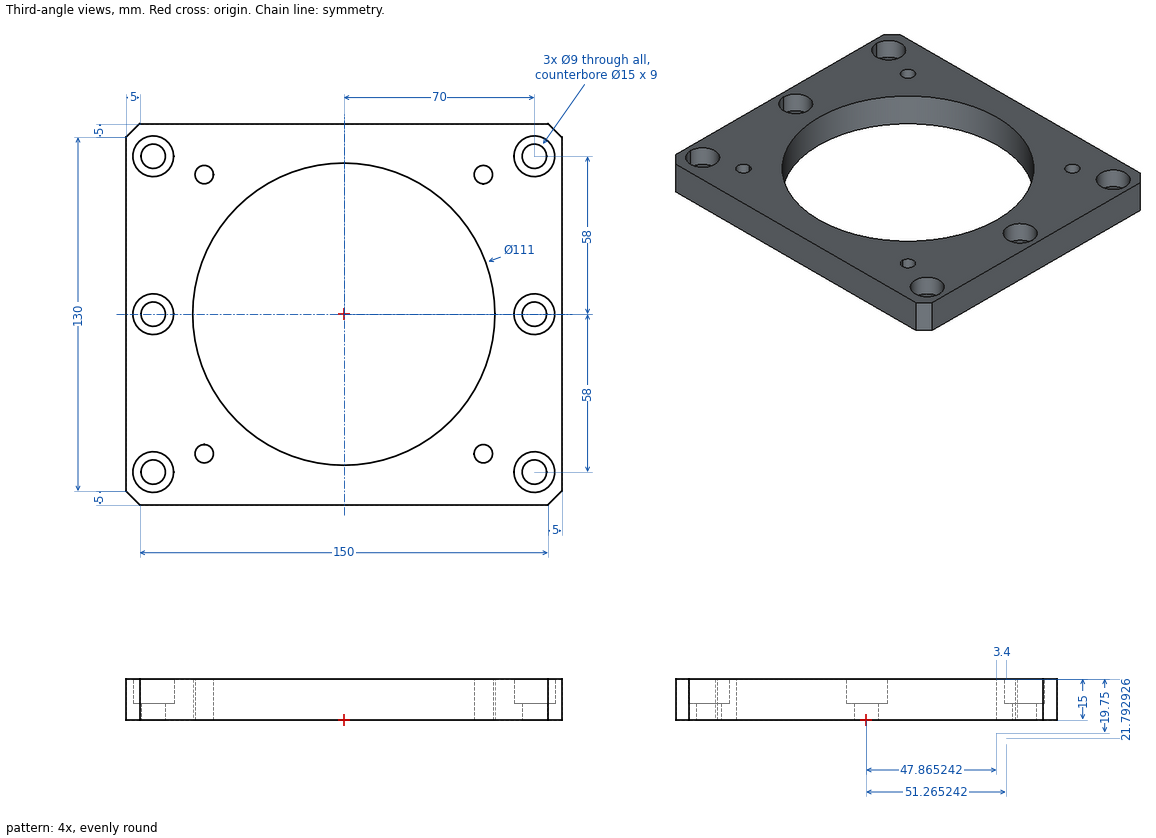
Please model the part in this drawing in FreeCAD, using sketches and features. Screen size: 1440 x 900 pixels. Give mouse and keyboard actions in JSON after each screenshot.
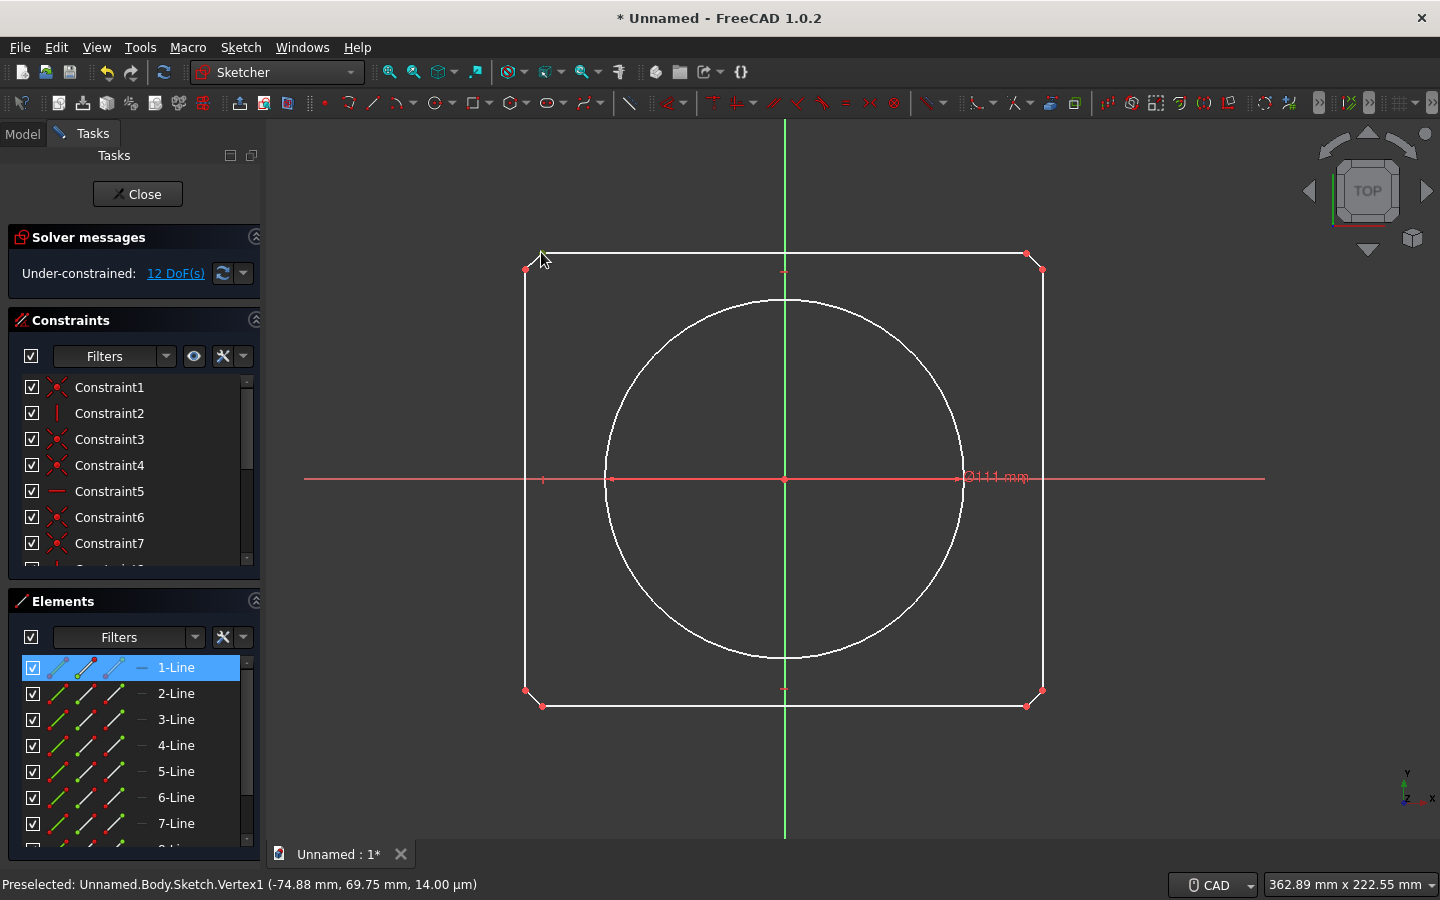
{"action": "left_click", "coordinate": [542, 706]}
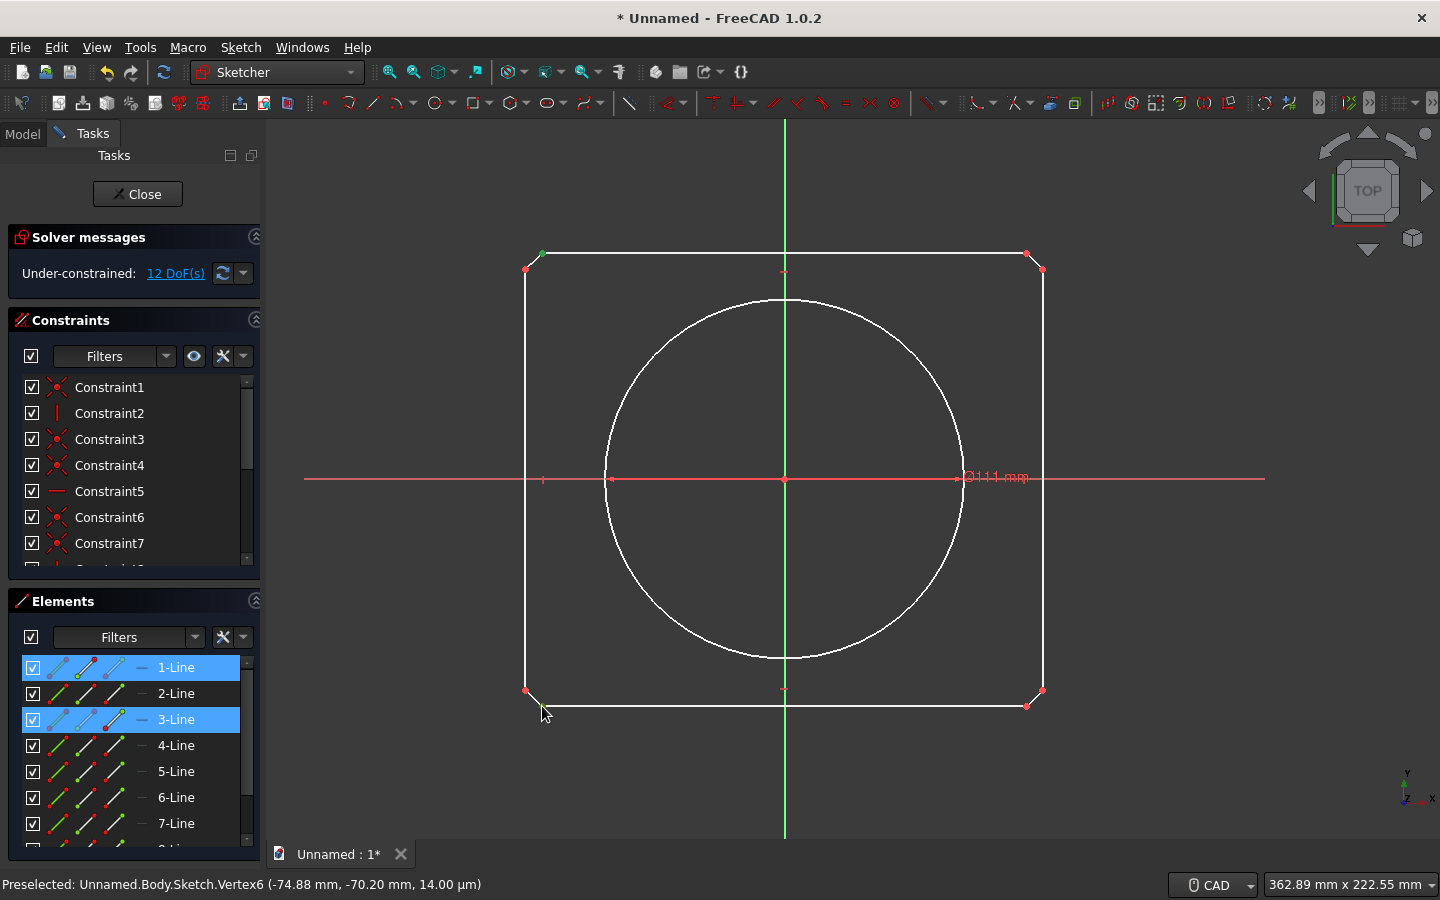
{"action": "left_click", "coordinate": [364, 479]}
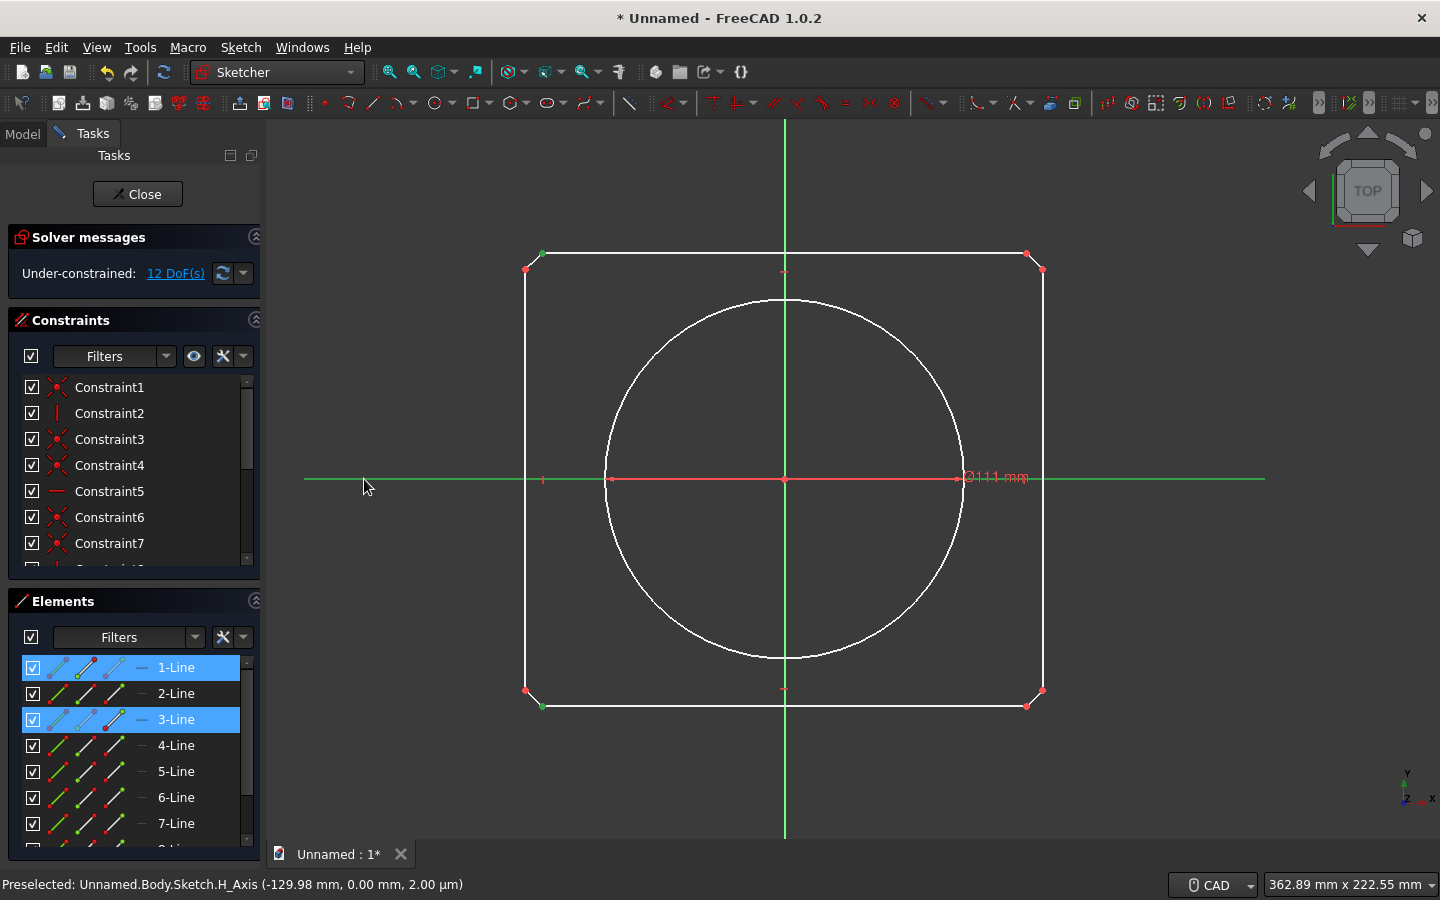
{"action": "left_click", "coordinate": [870, 104]}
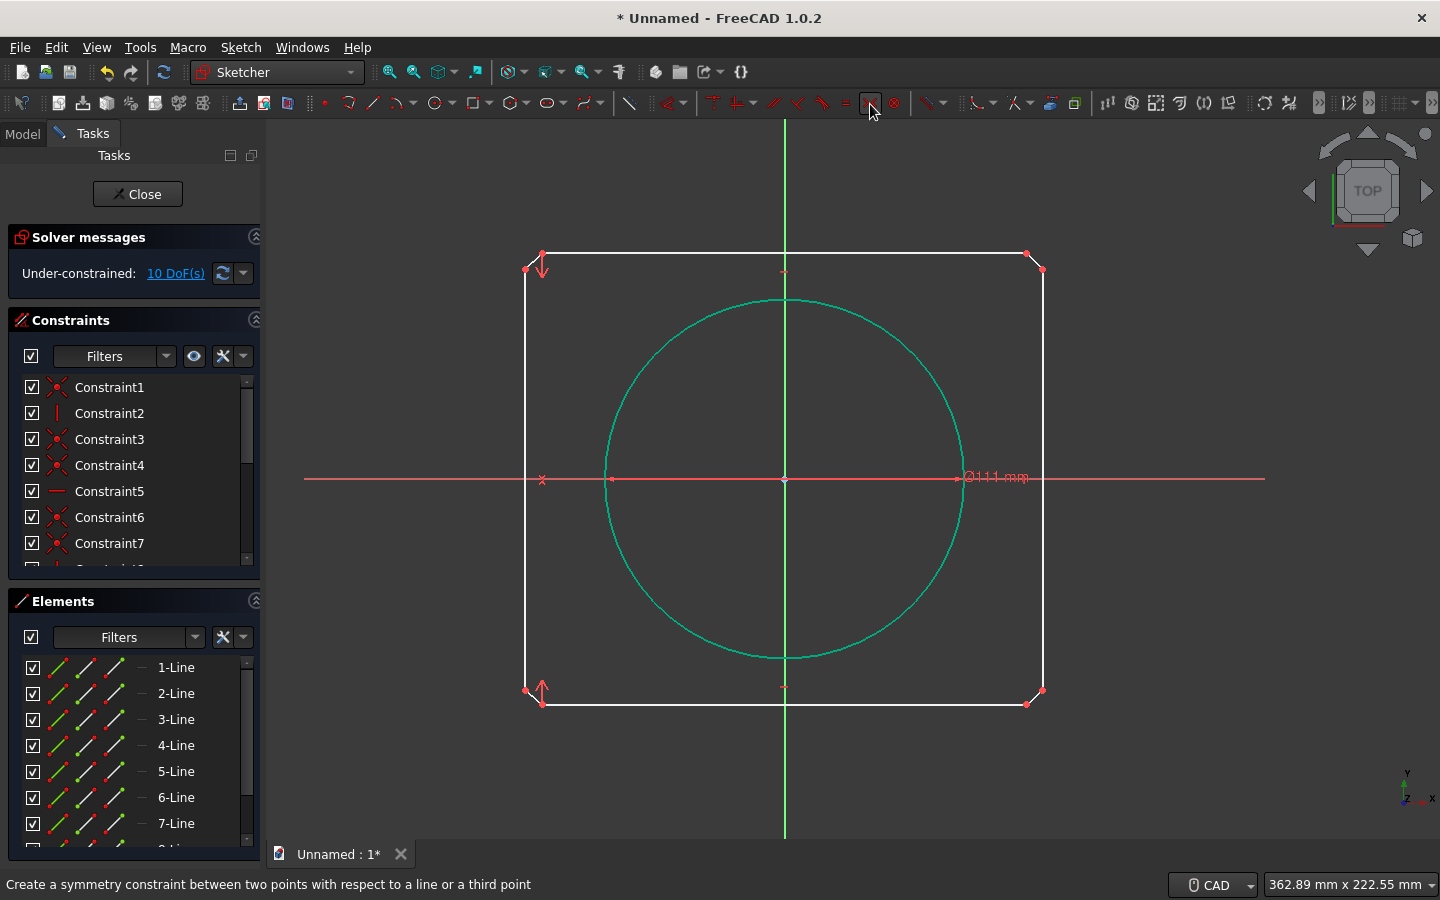
{"action": "left_click", "coordinate": [525, 690]}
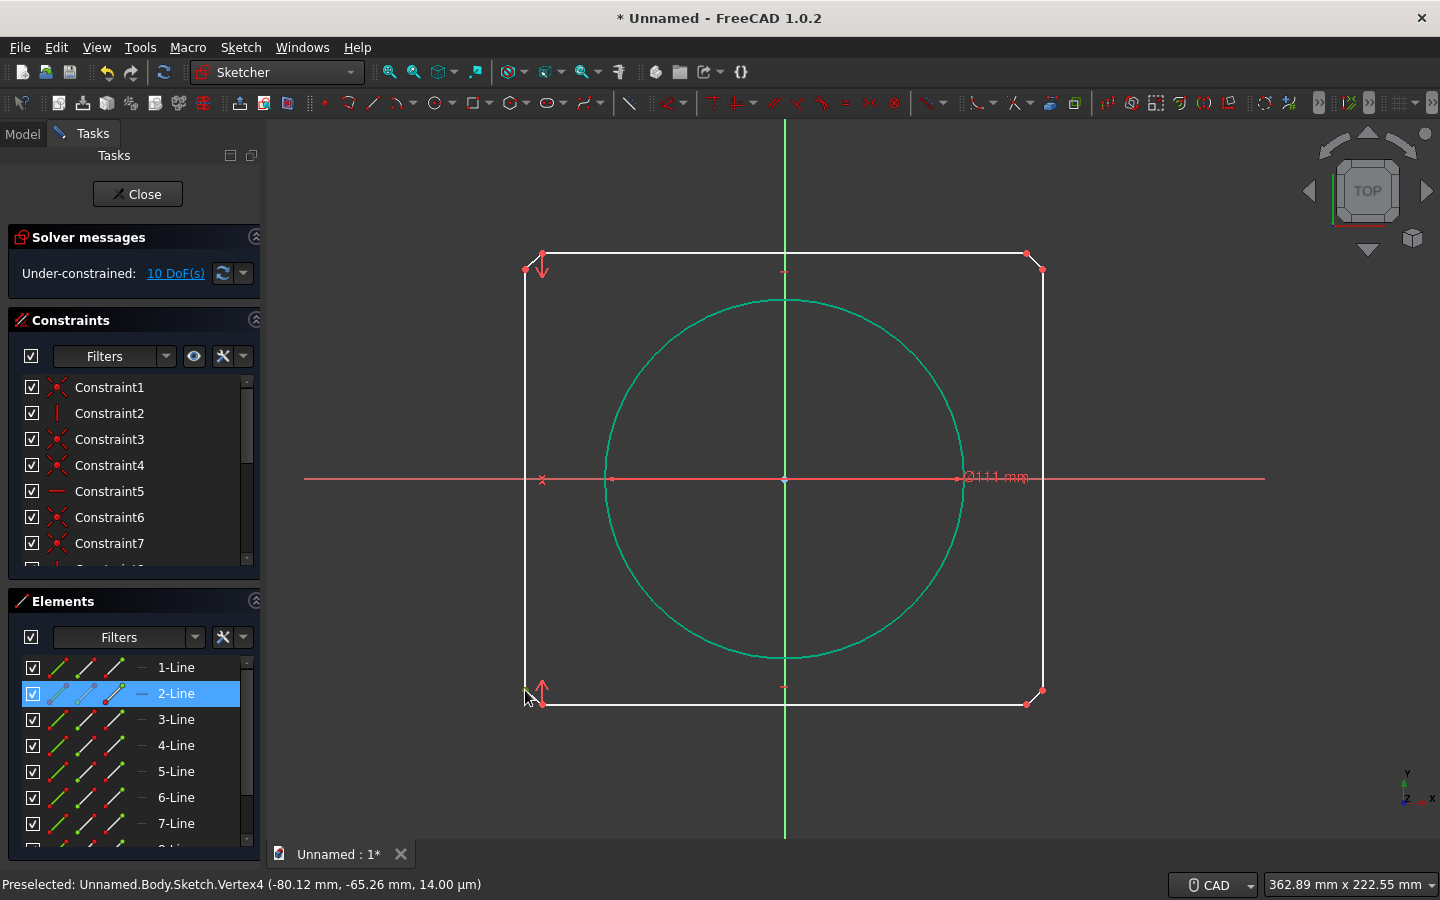
{"action": "left_click", "coordinate": [1043, 690]}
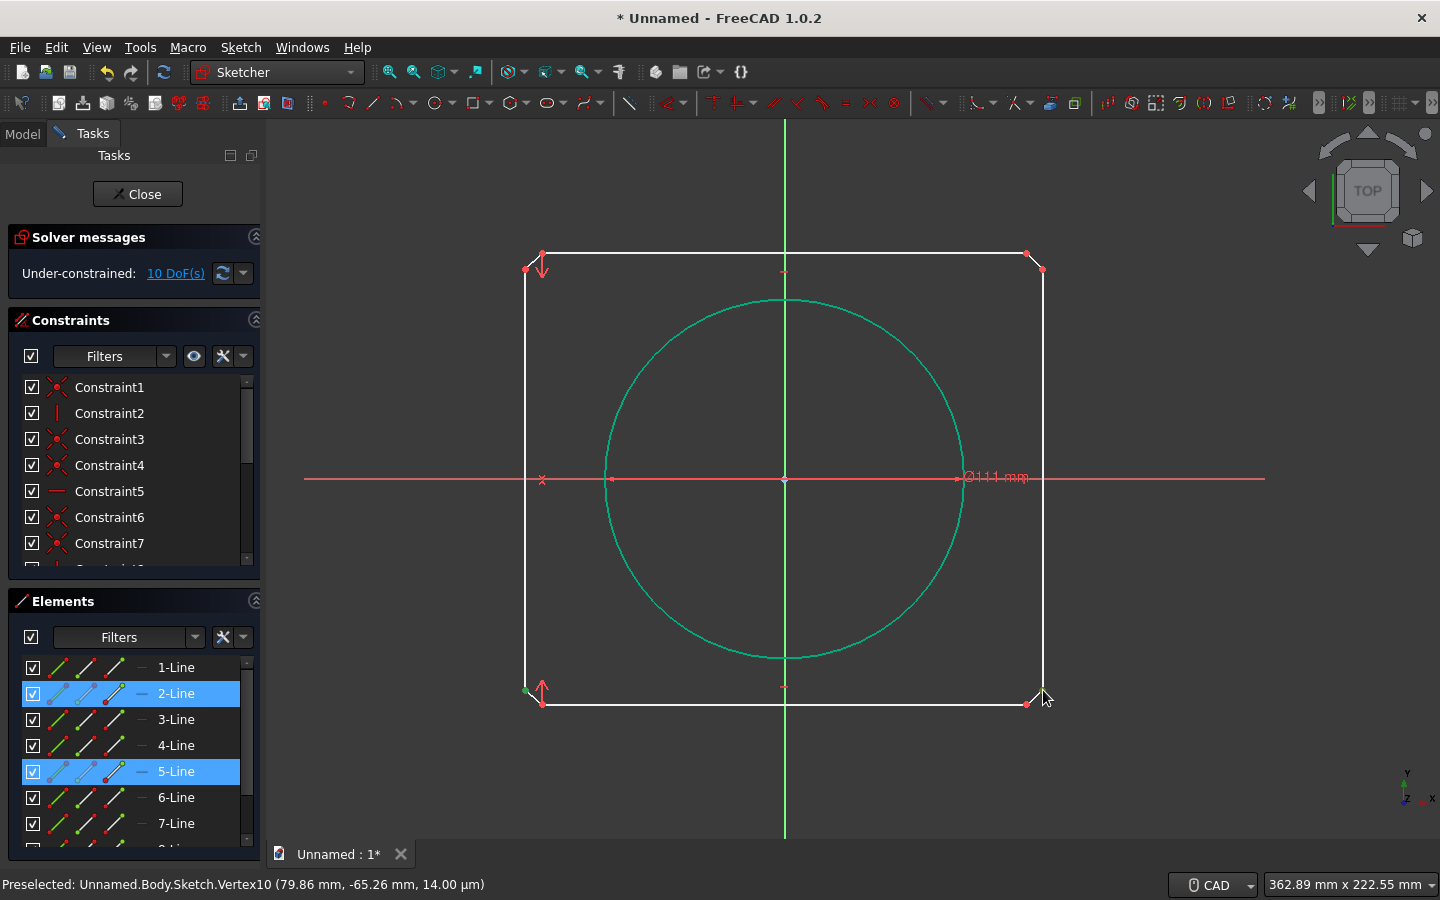
{"action": "left_click", "coordinate": [785, 764]}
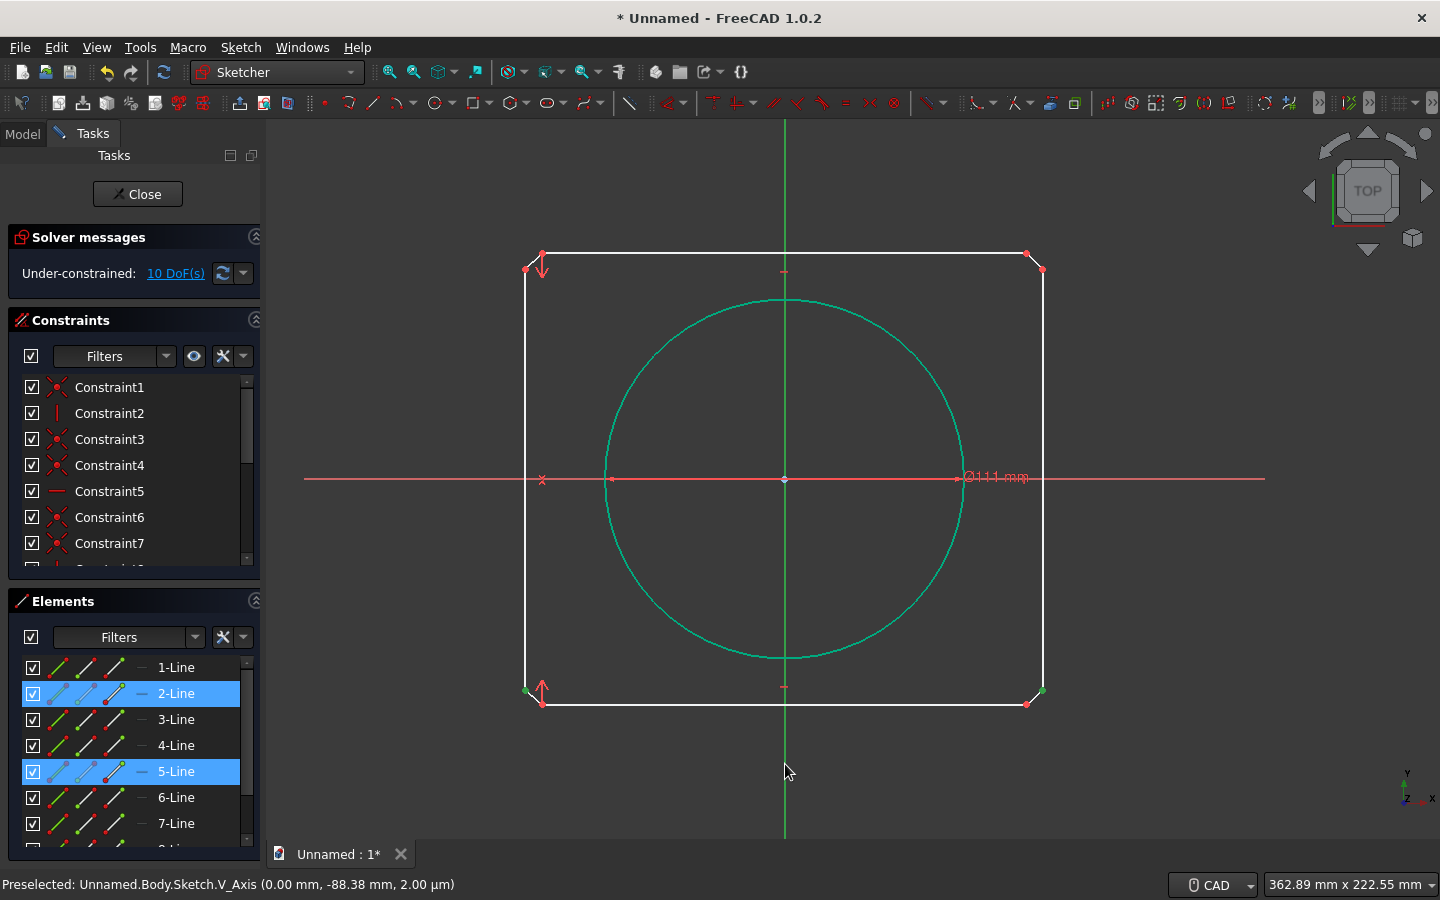
{"action": "left_click", "coordinate": [870, 104]}